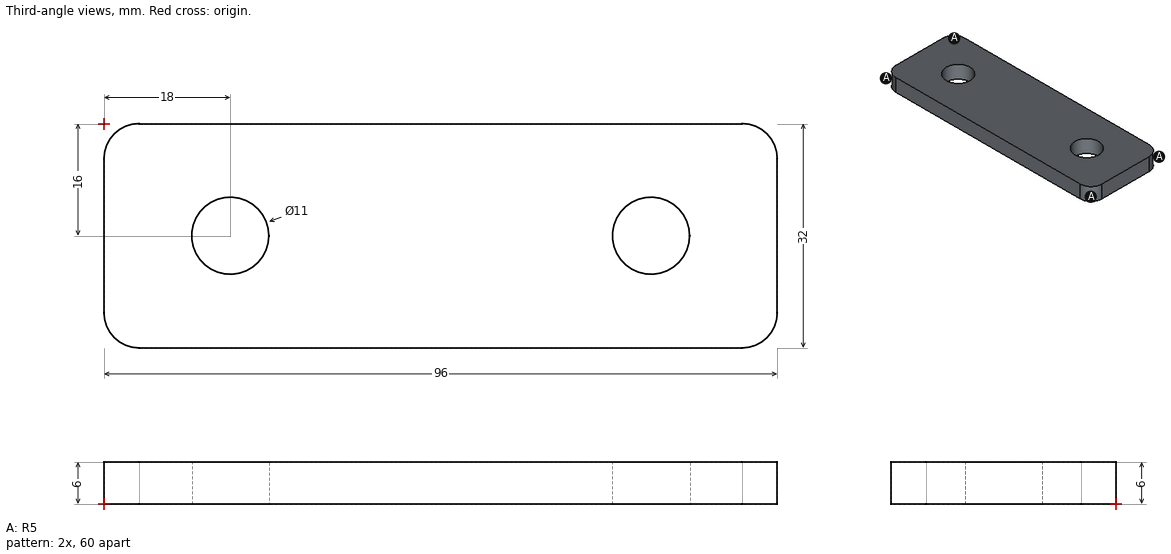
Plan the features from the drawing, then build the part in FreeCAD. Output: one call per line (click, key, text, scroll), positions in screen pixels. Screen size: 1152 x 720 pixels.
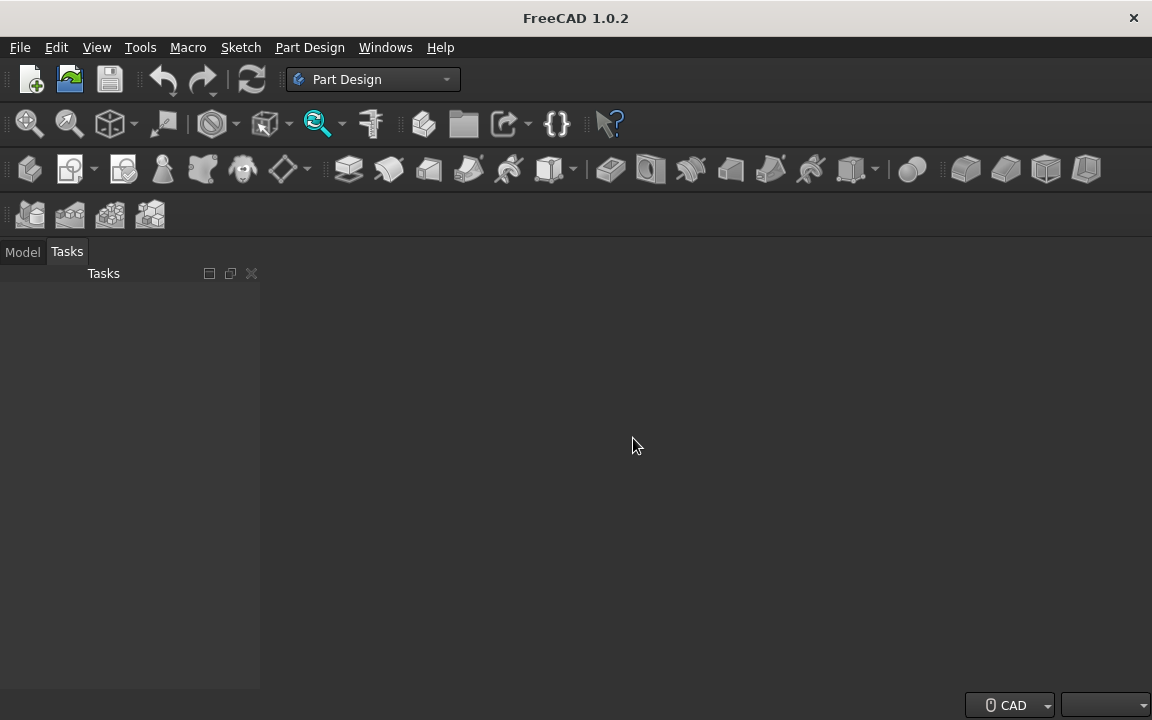
click(30, 80)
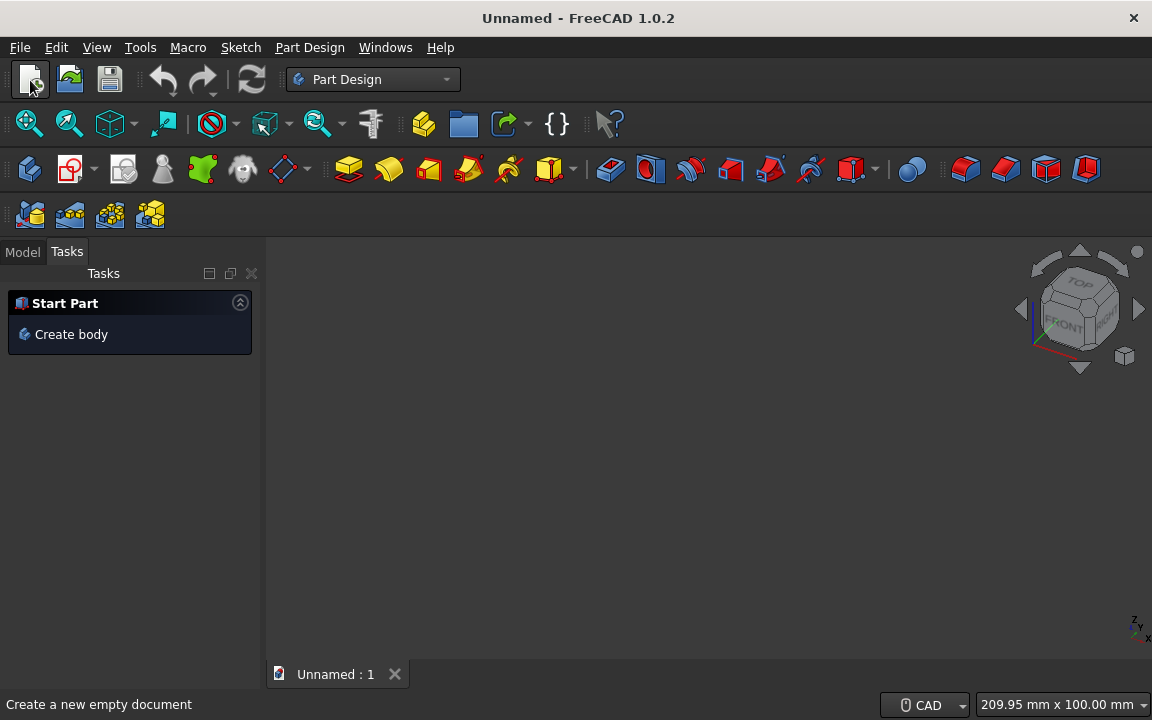
click(70, 170)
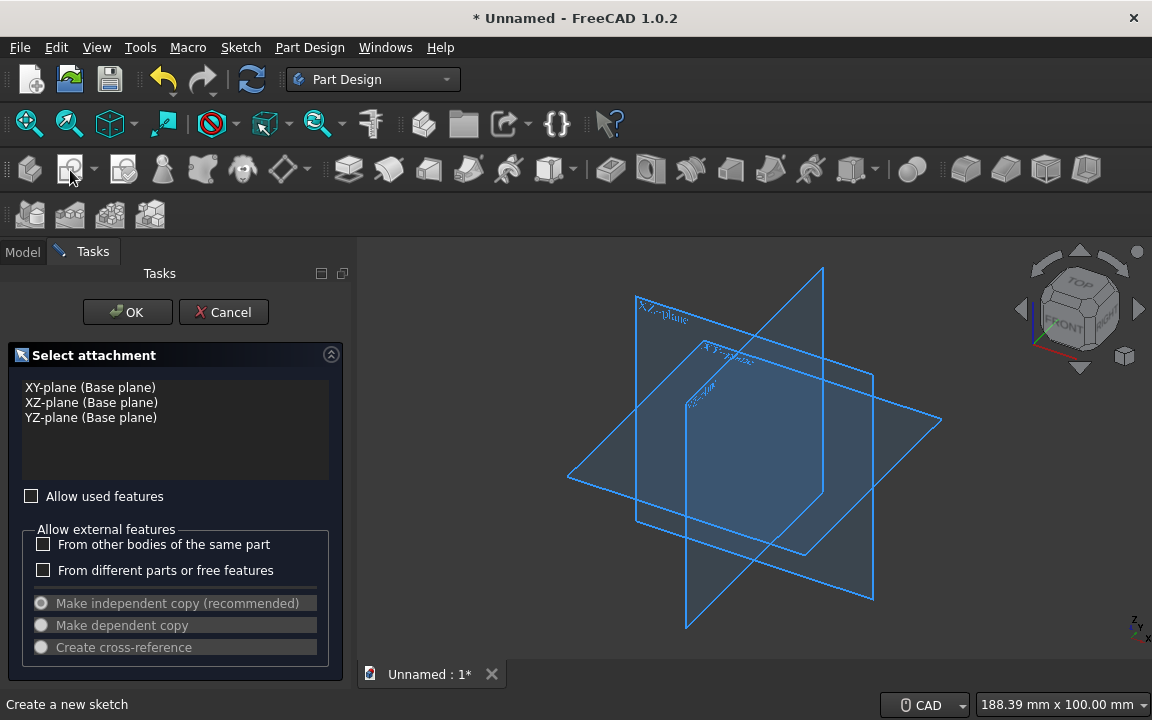
click(82, 388)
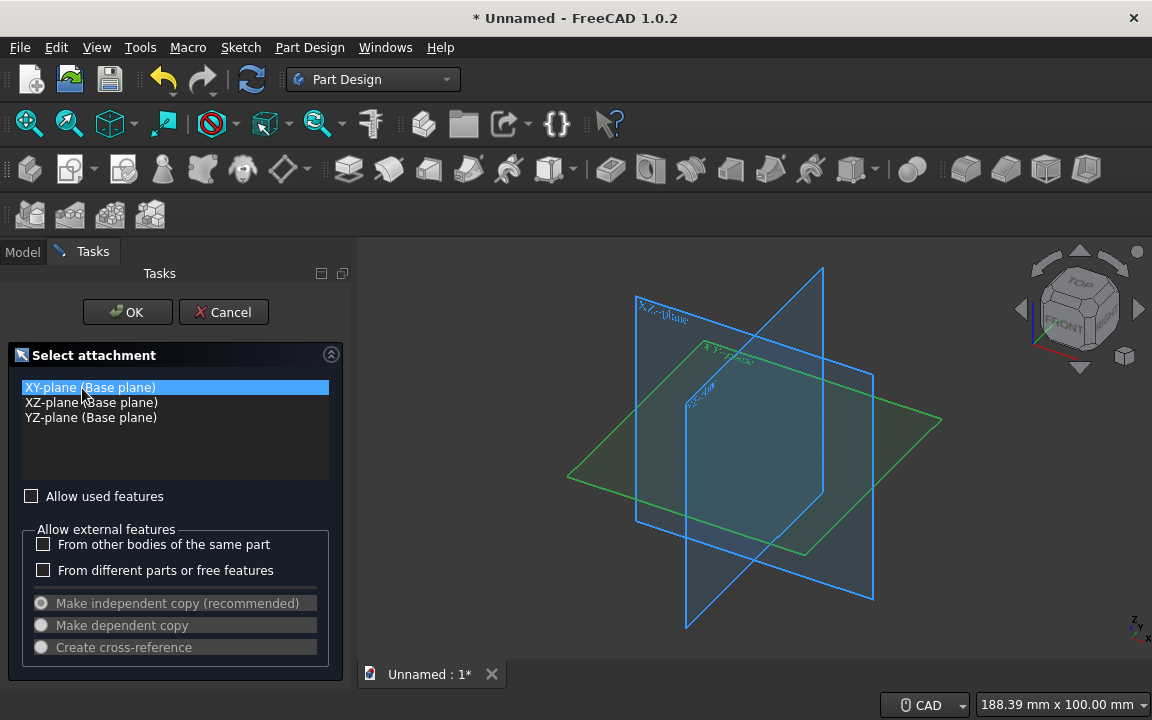
click(128, 312)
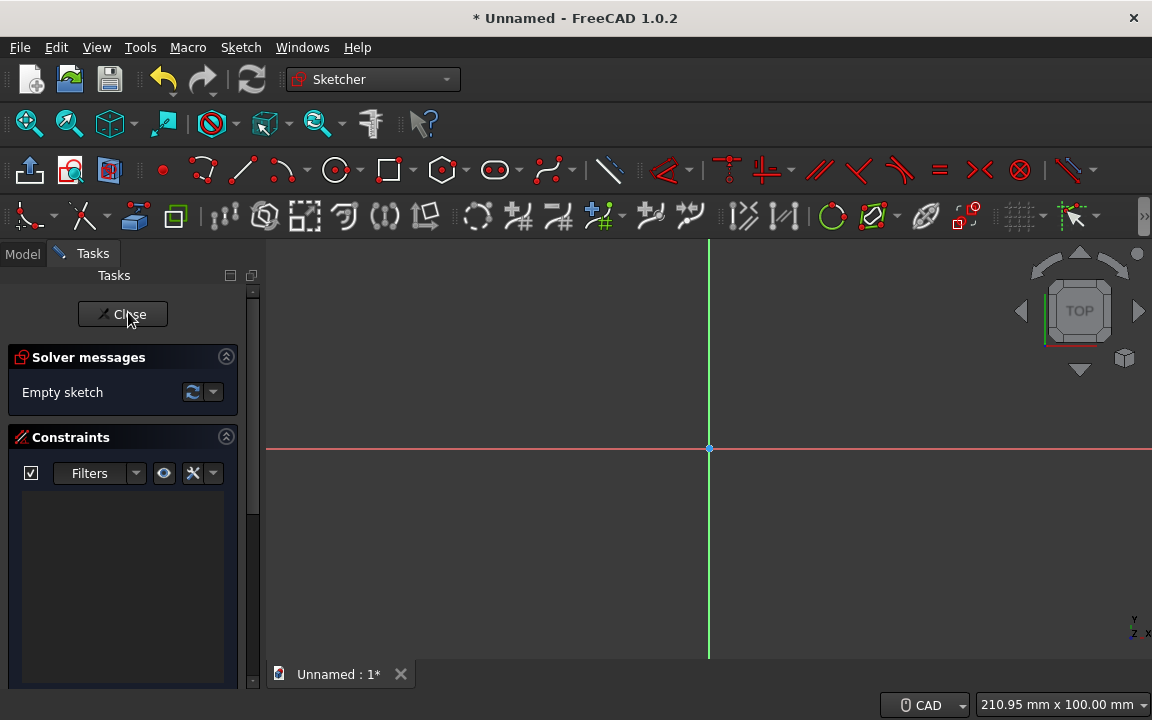
scroll(294, 312, down, 2)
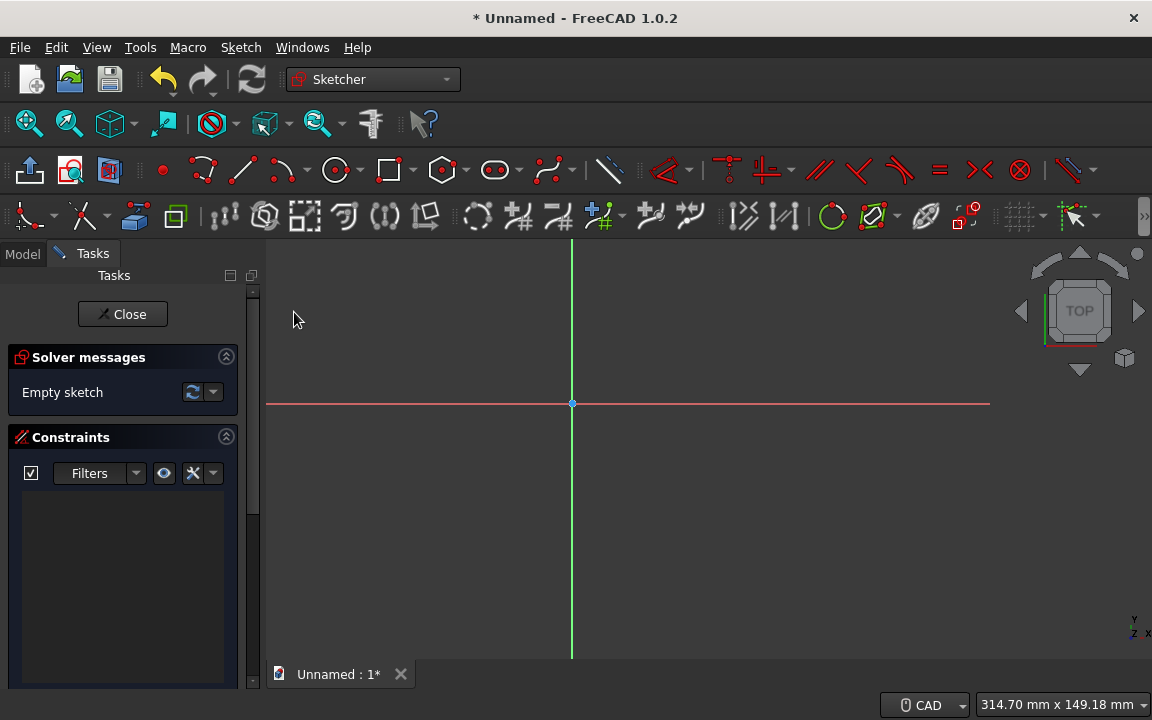
scroll(789, 449, up, 3)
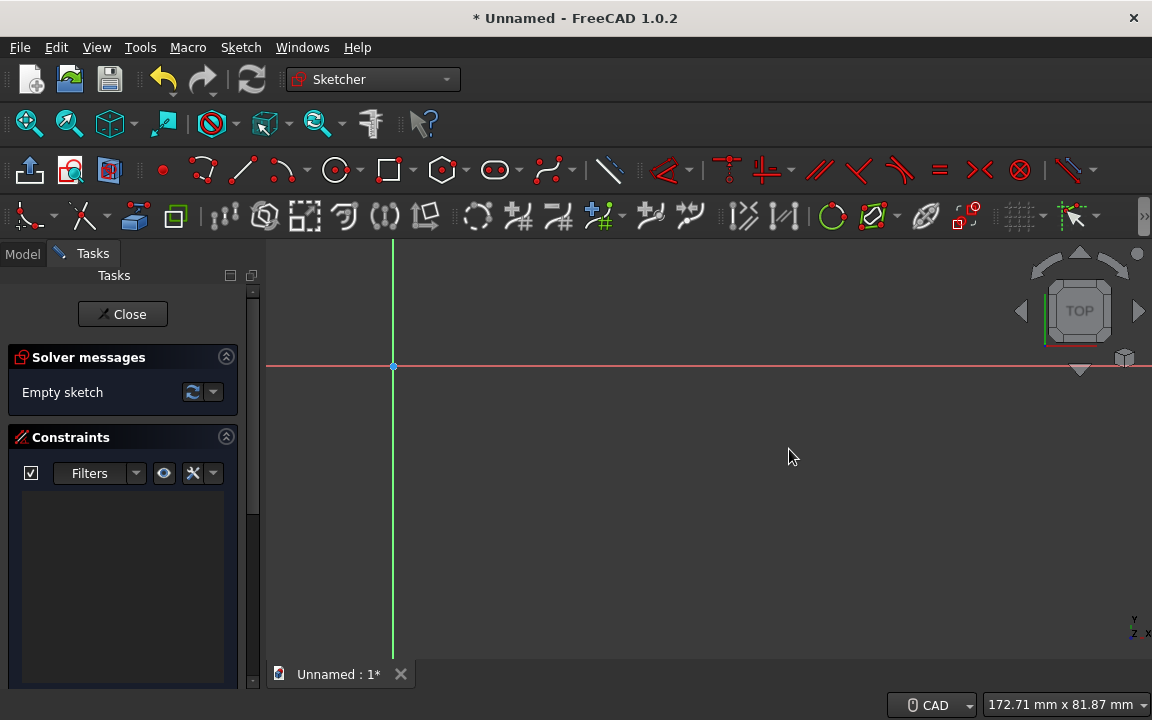
key(g)
key(r)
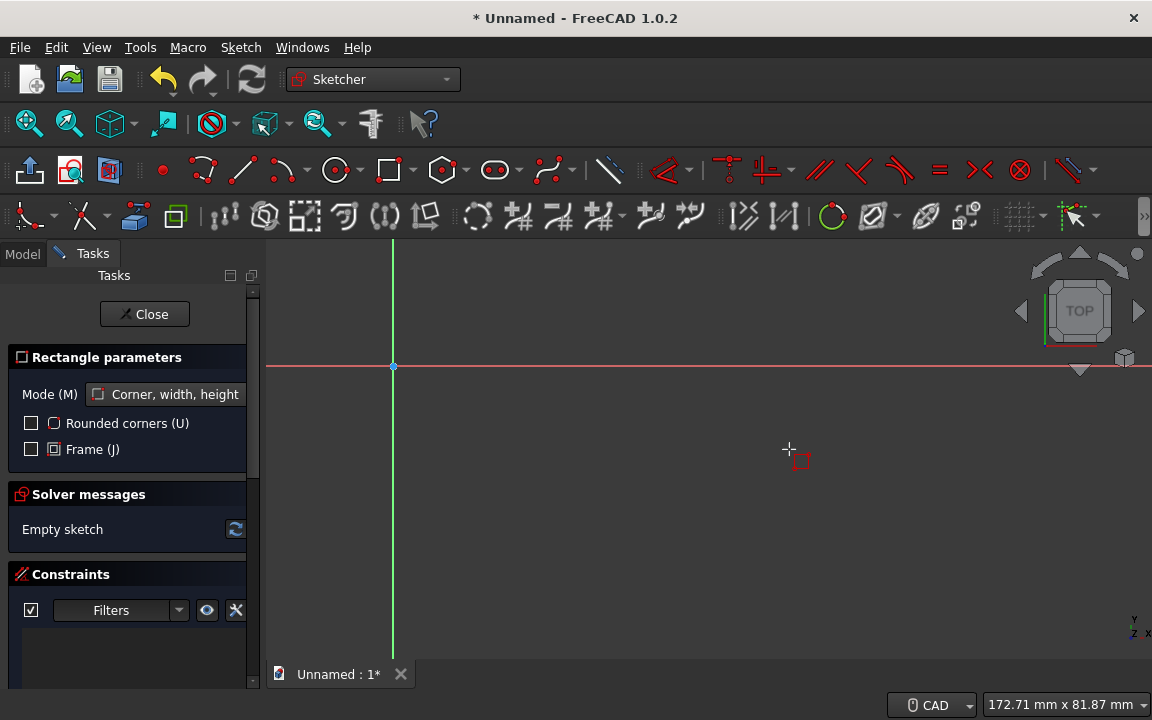
click(393, 366)
move(886, 531)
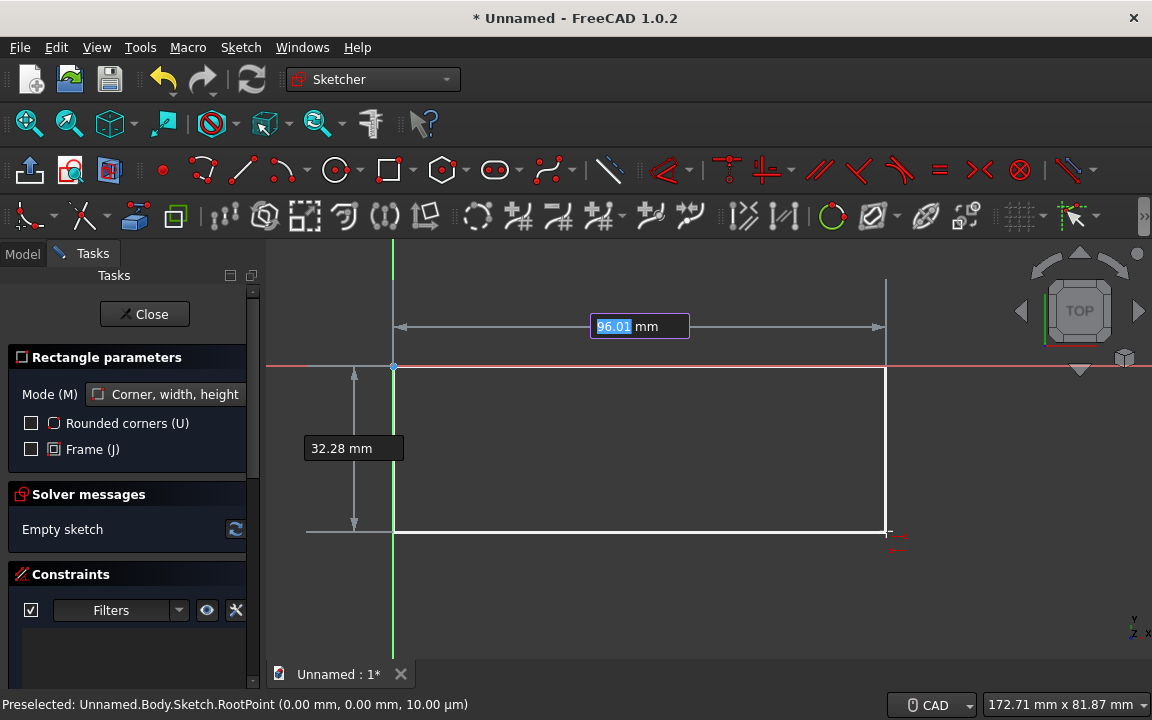
text(96)
key(Tab)
text(32)
key(Return)
key(Escape)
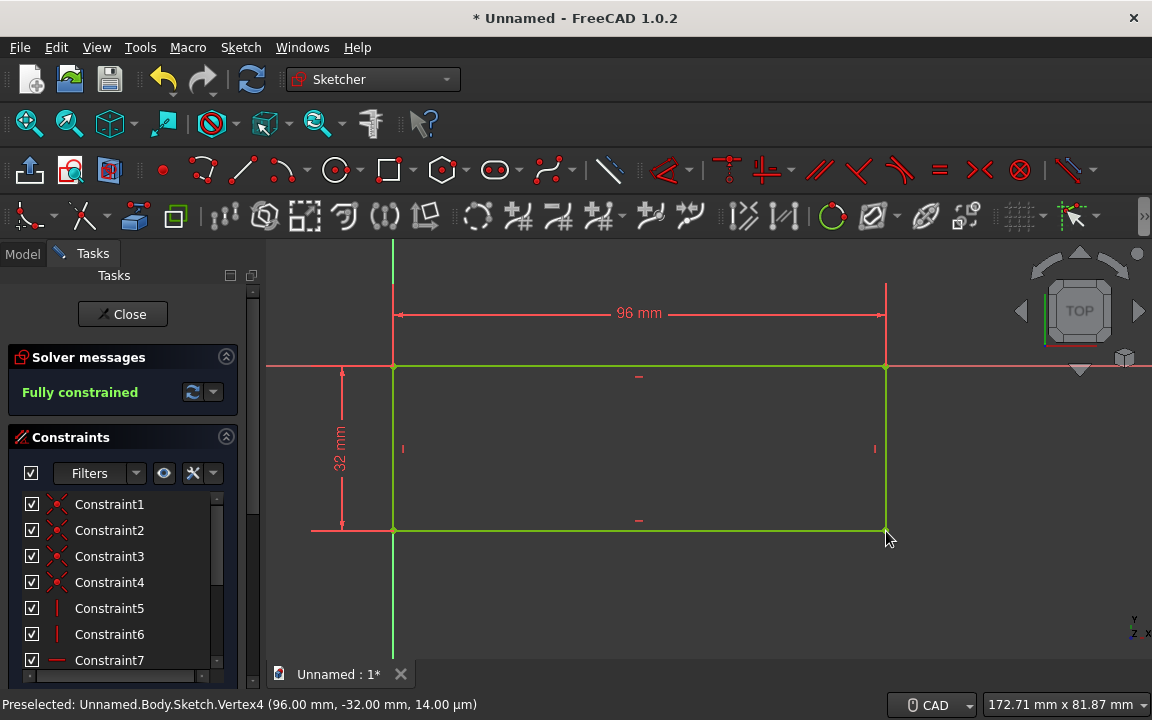
click(123, 314)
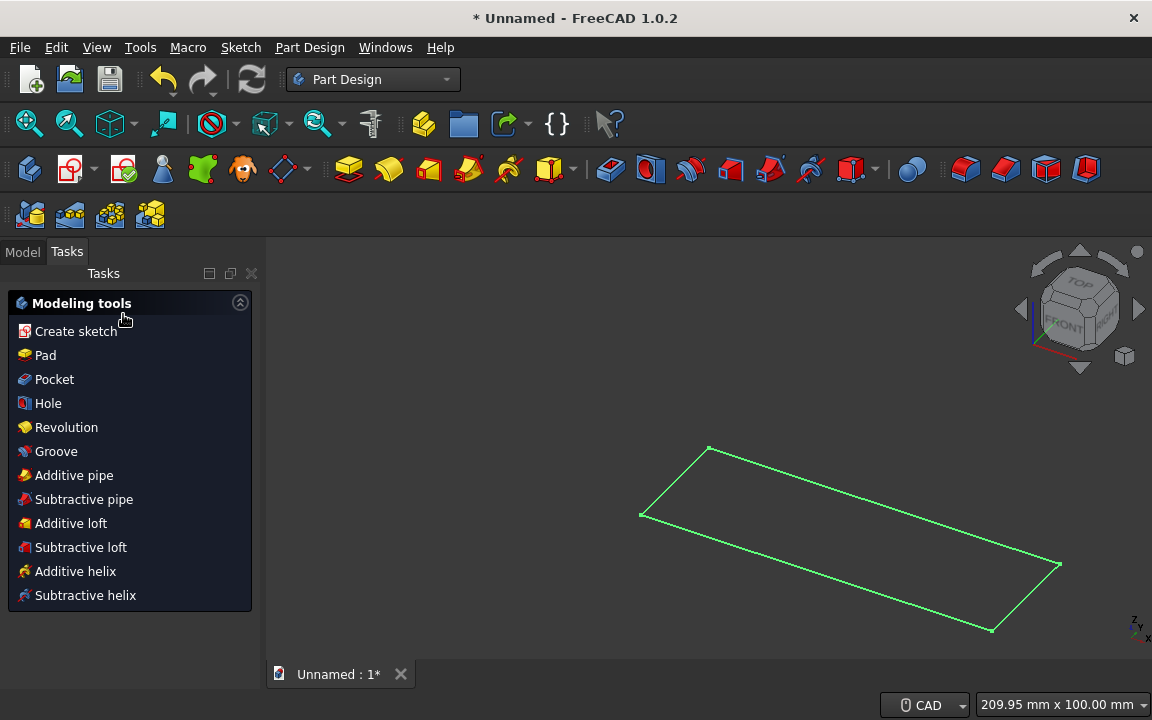
click(350, 170)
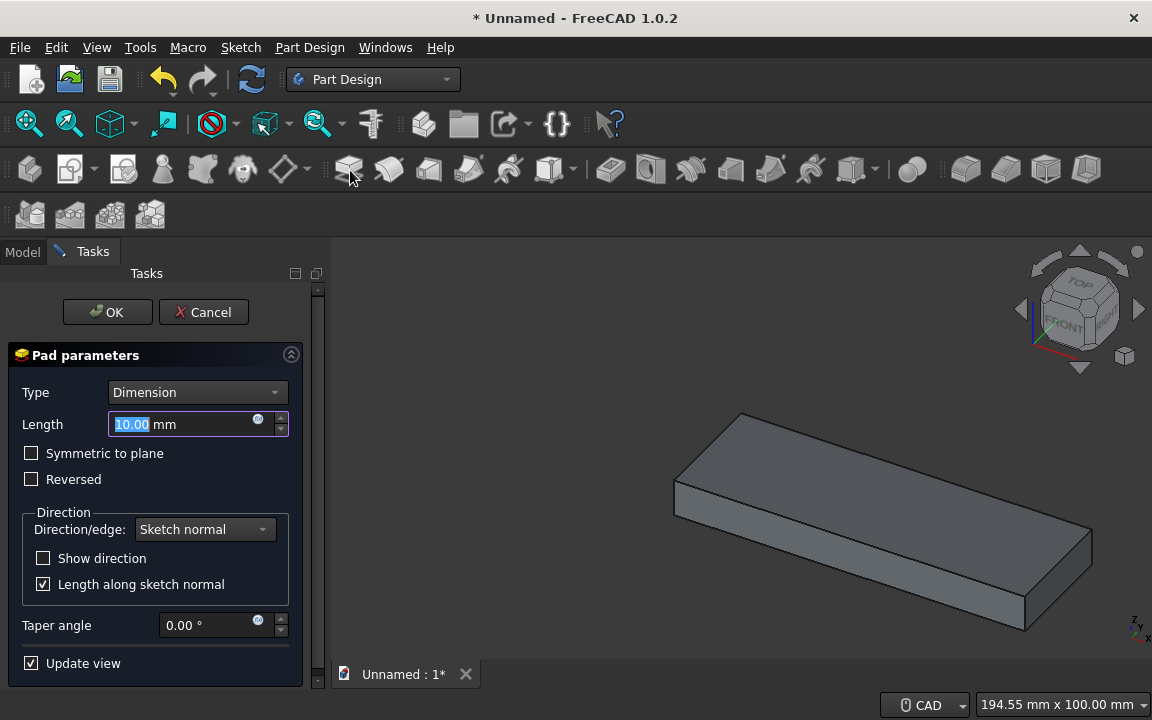
text(6)
key(Tab)